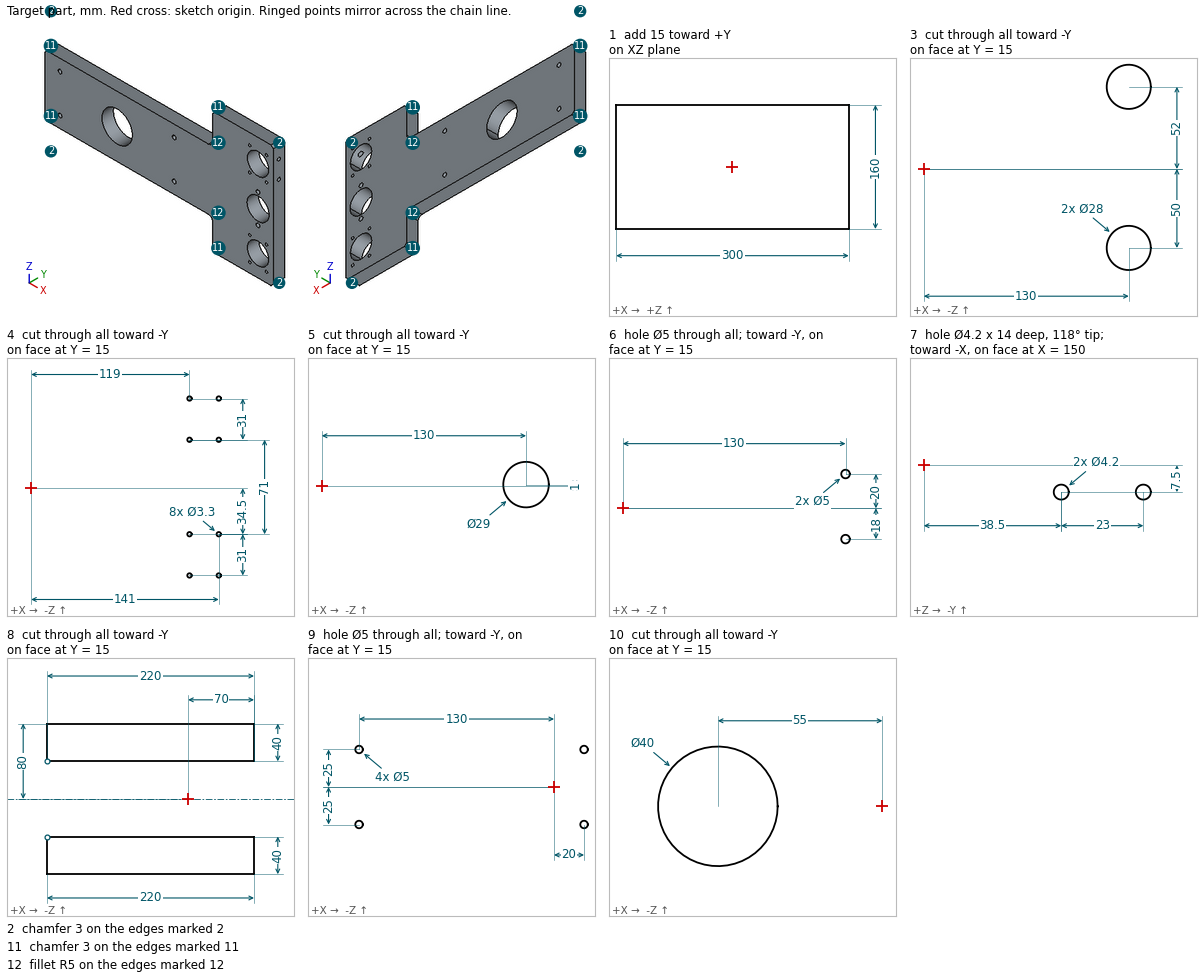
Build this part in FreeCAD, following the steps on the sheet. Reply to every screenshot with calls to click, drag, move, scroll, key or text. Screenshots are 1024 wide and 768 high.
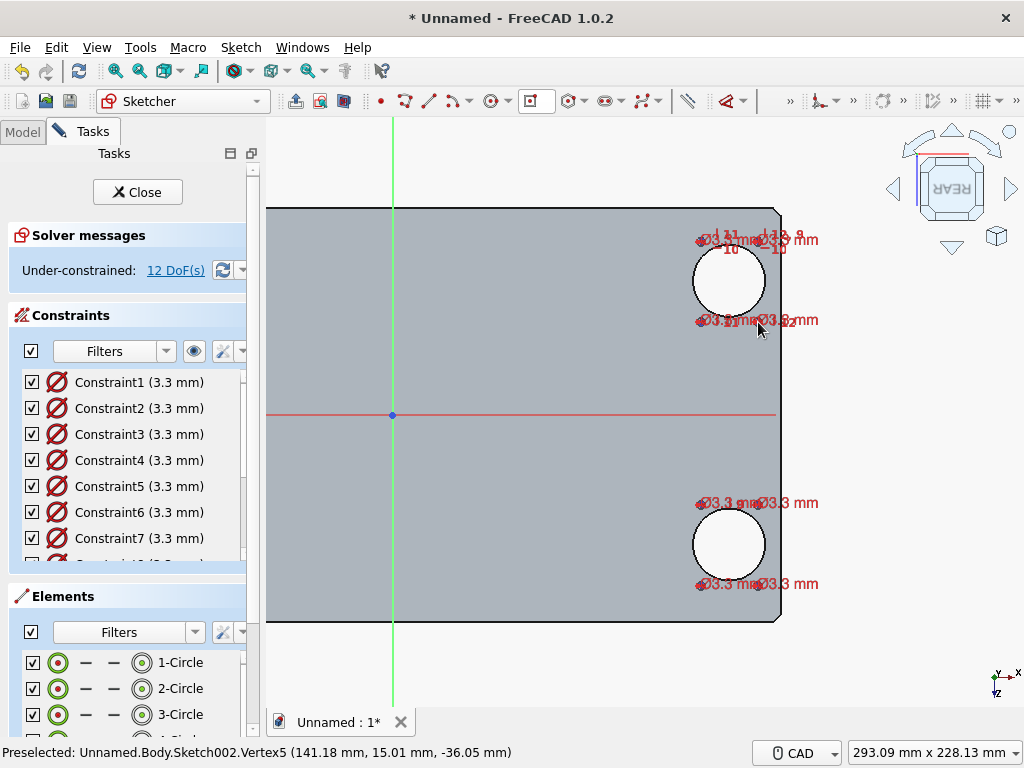
click(701, 322)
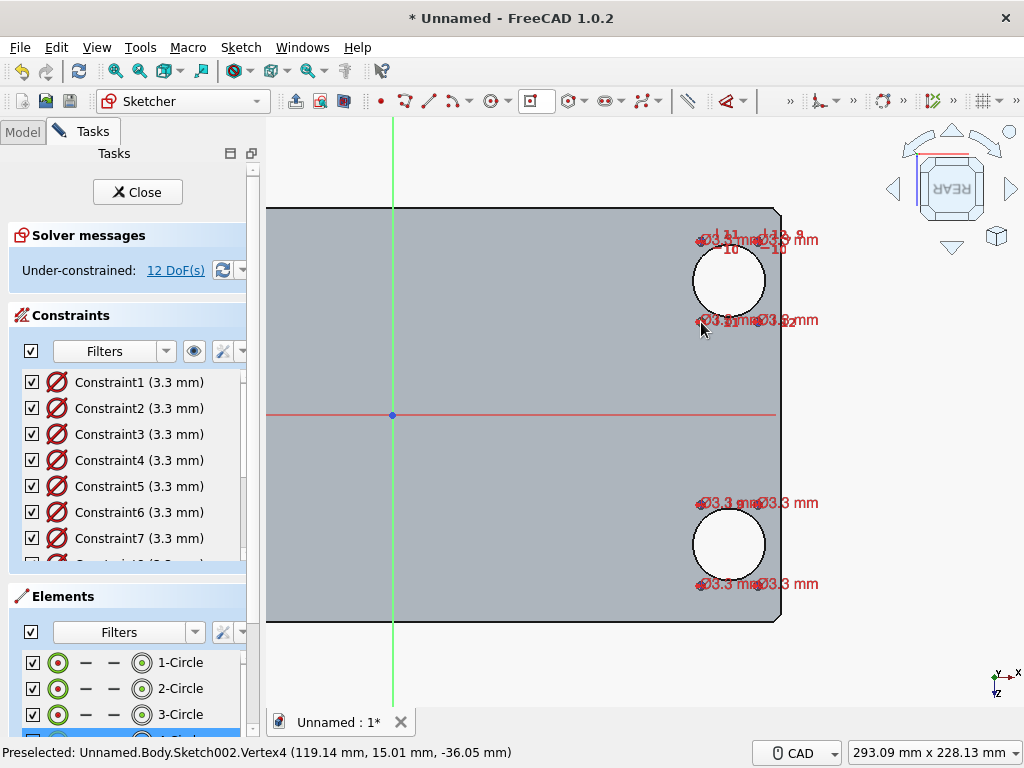
click(758, 322)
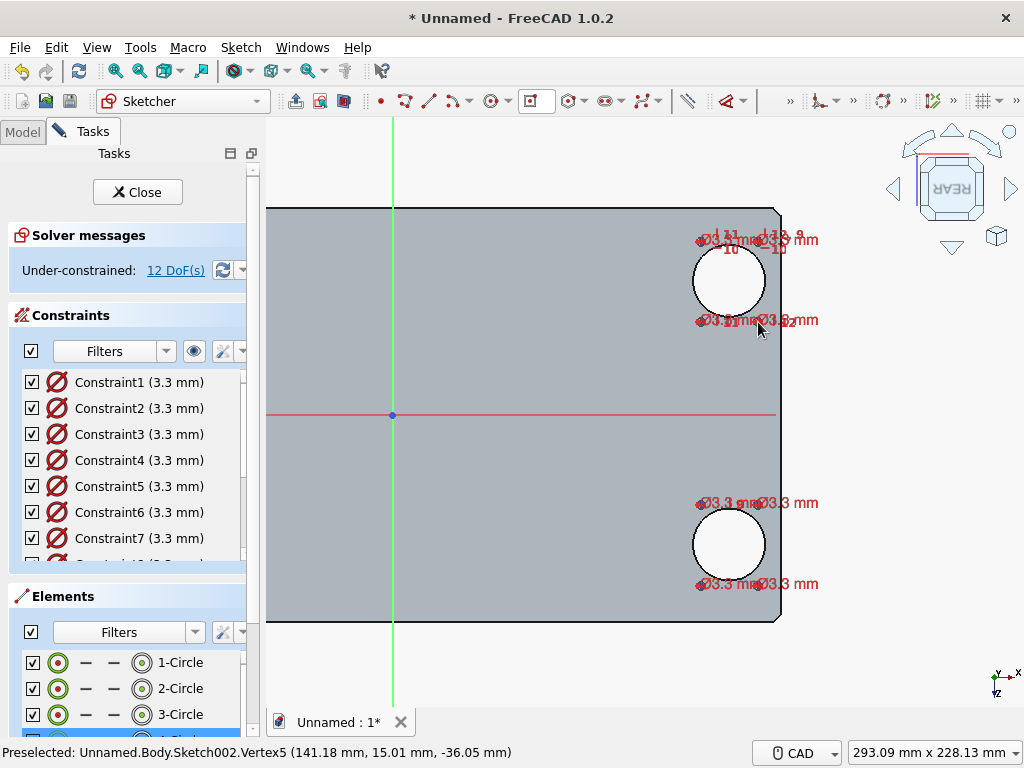
key(h)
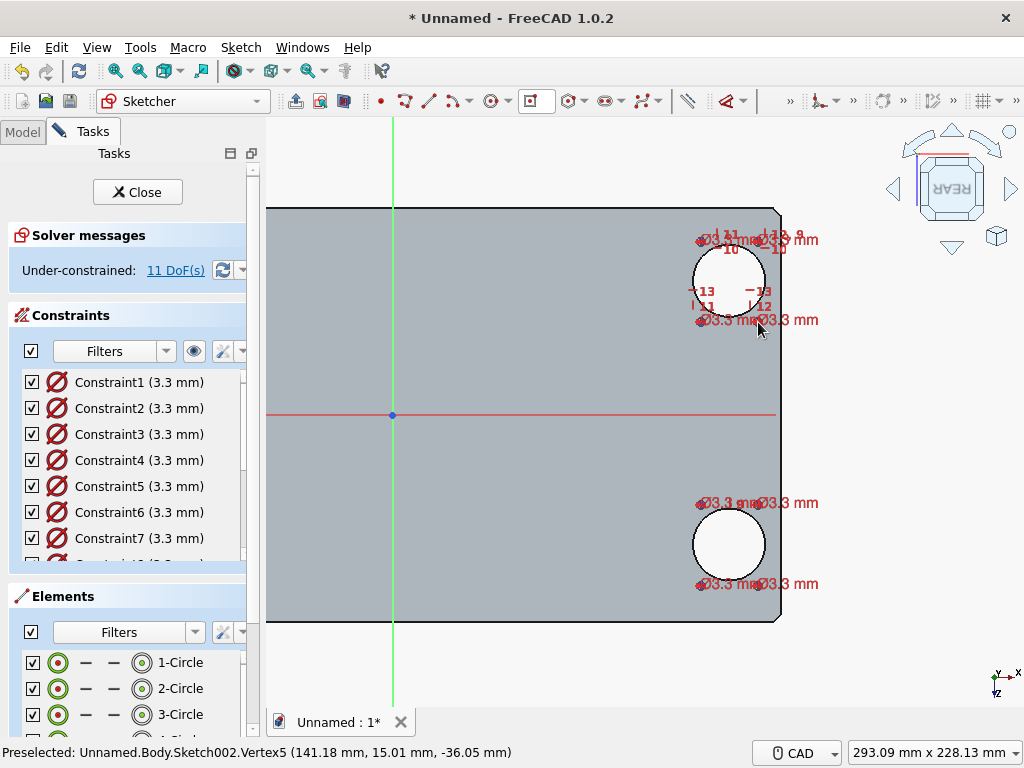
click(701, 322)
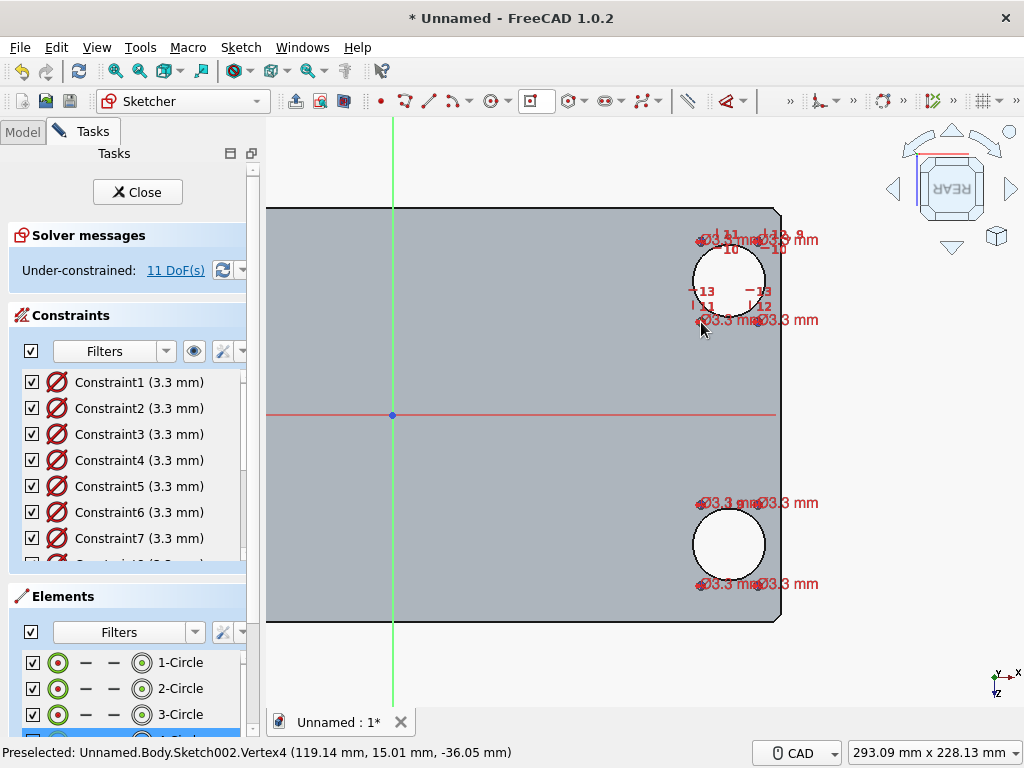
click(701, 505)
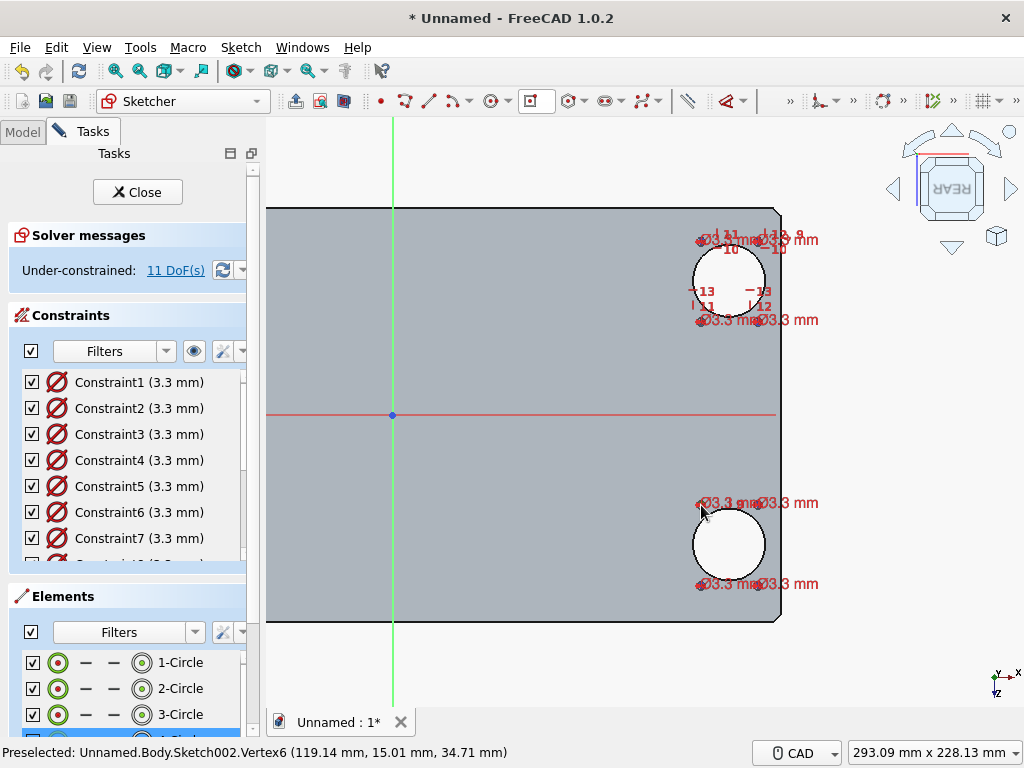
key(v)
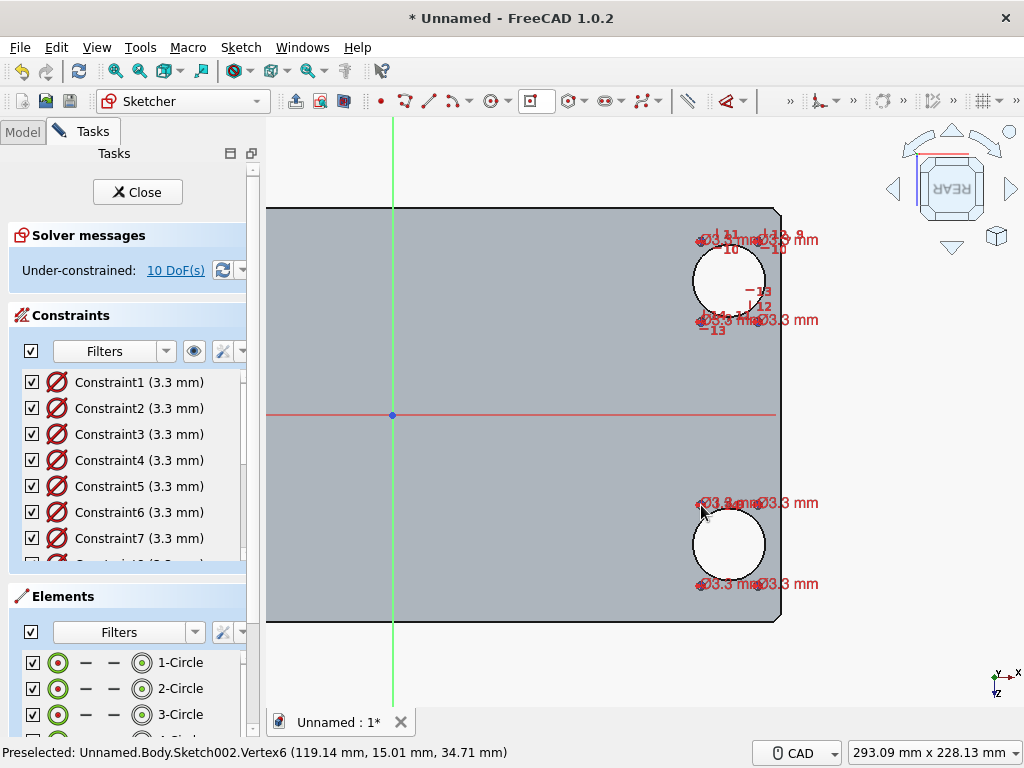
click(758, 505)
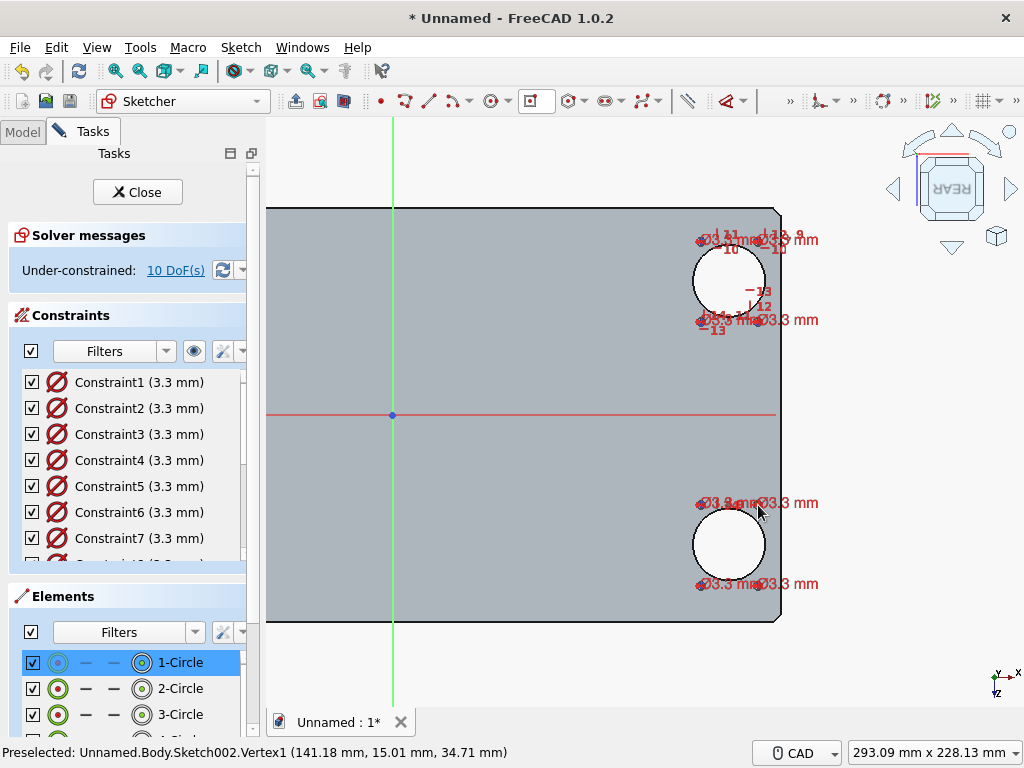
click(701, 505)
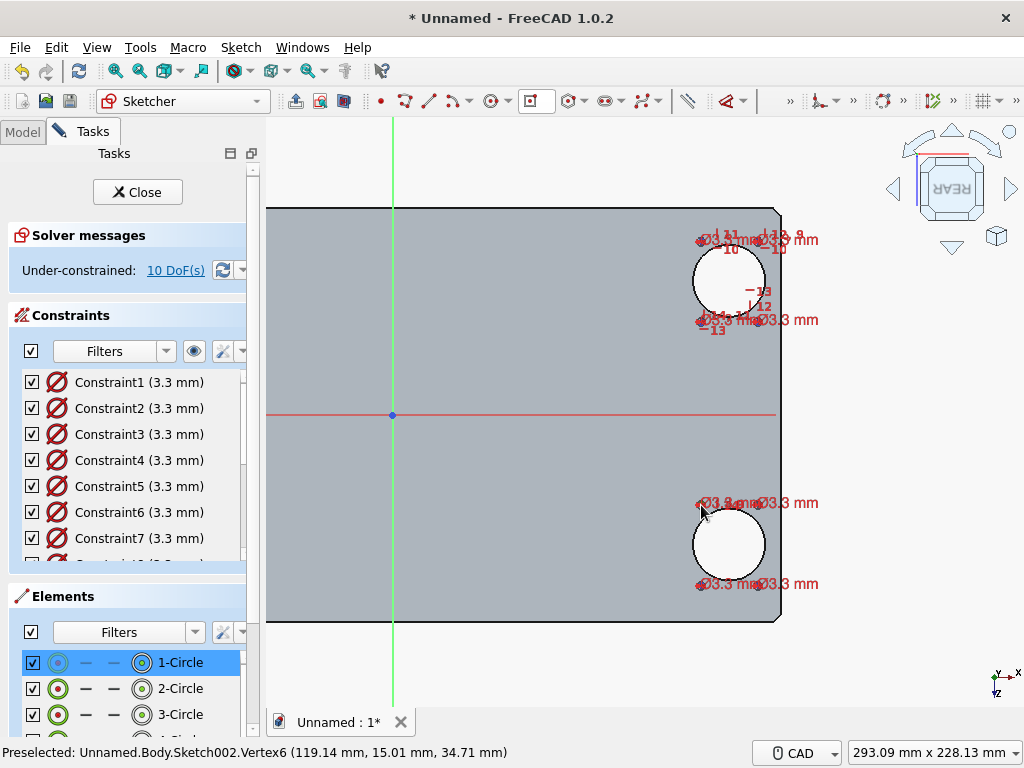
key(h)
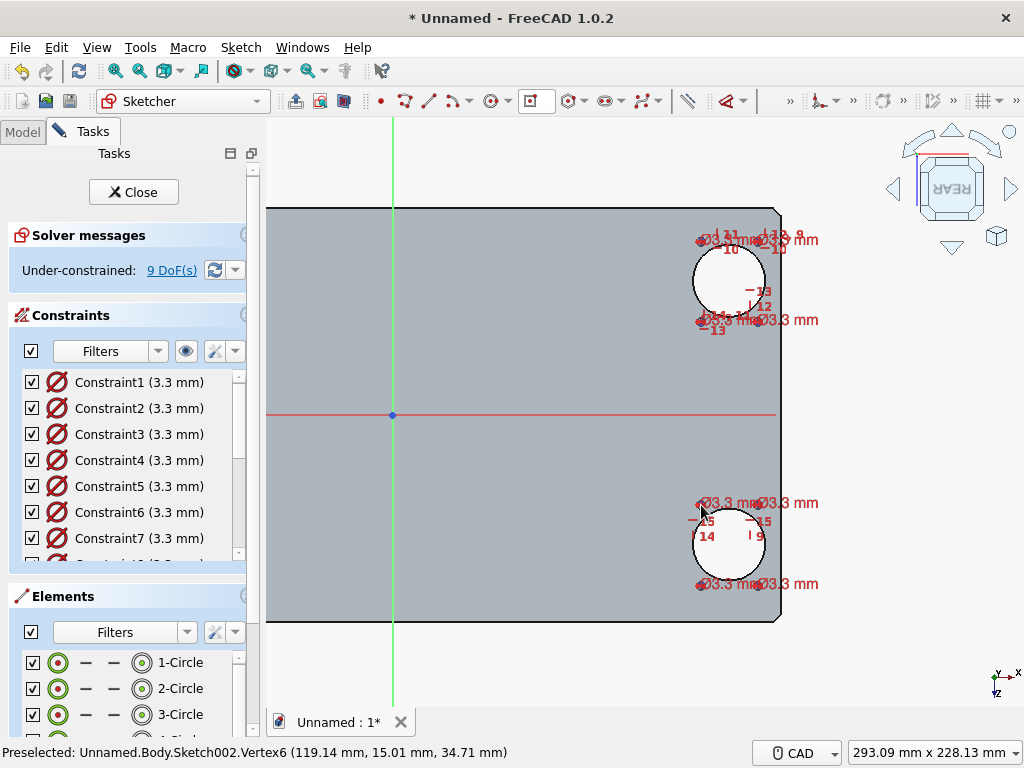
click(701, 505)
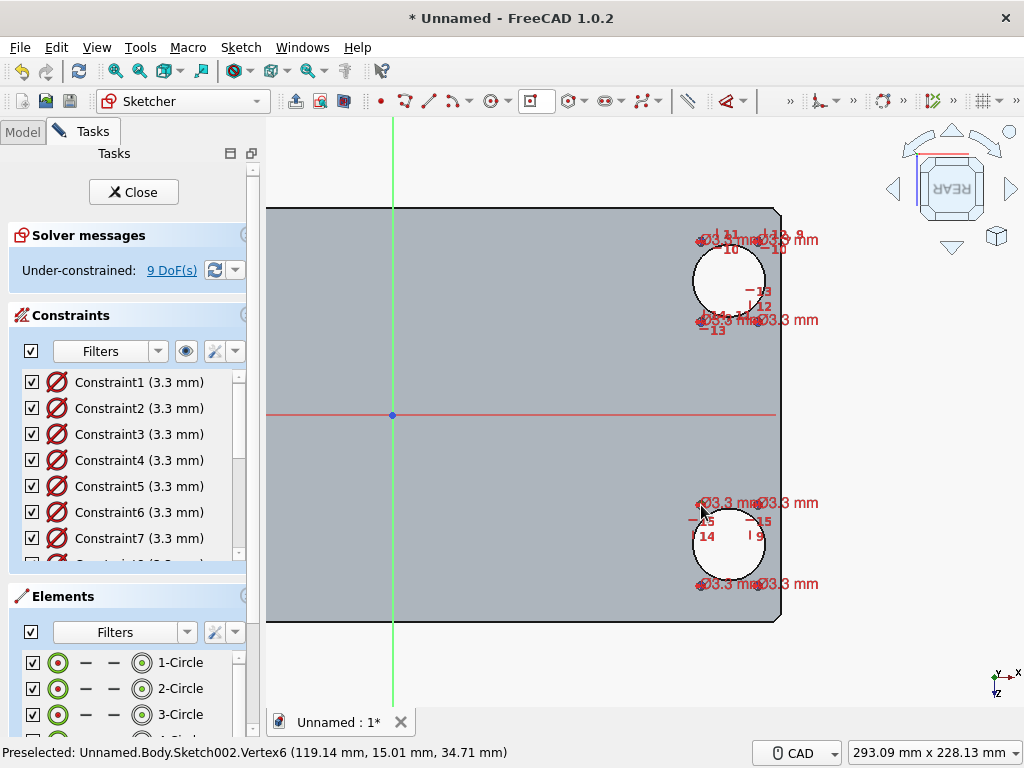
click(701, 586)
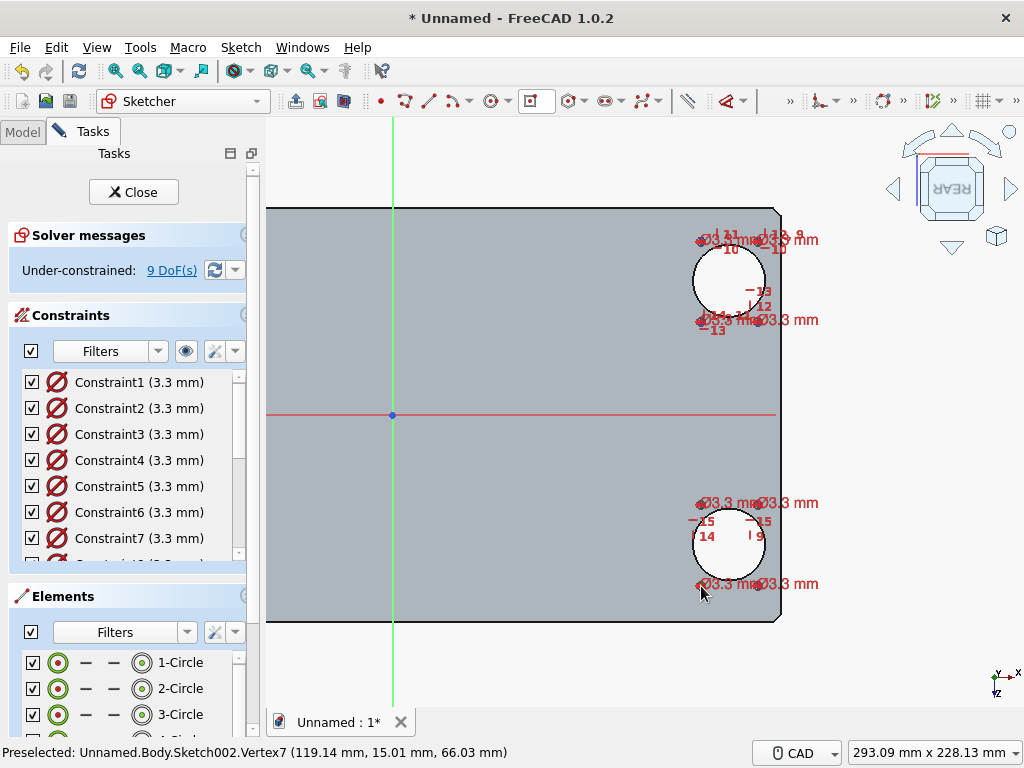
key(v)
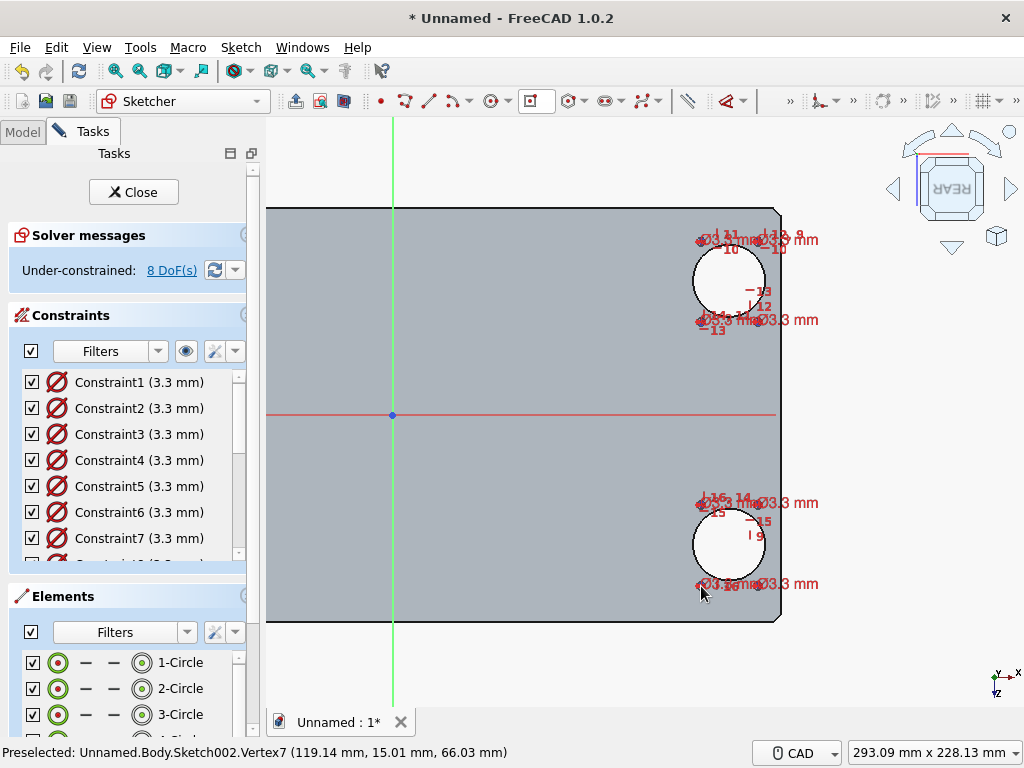
click(758, 505)